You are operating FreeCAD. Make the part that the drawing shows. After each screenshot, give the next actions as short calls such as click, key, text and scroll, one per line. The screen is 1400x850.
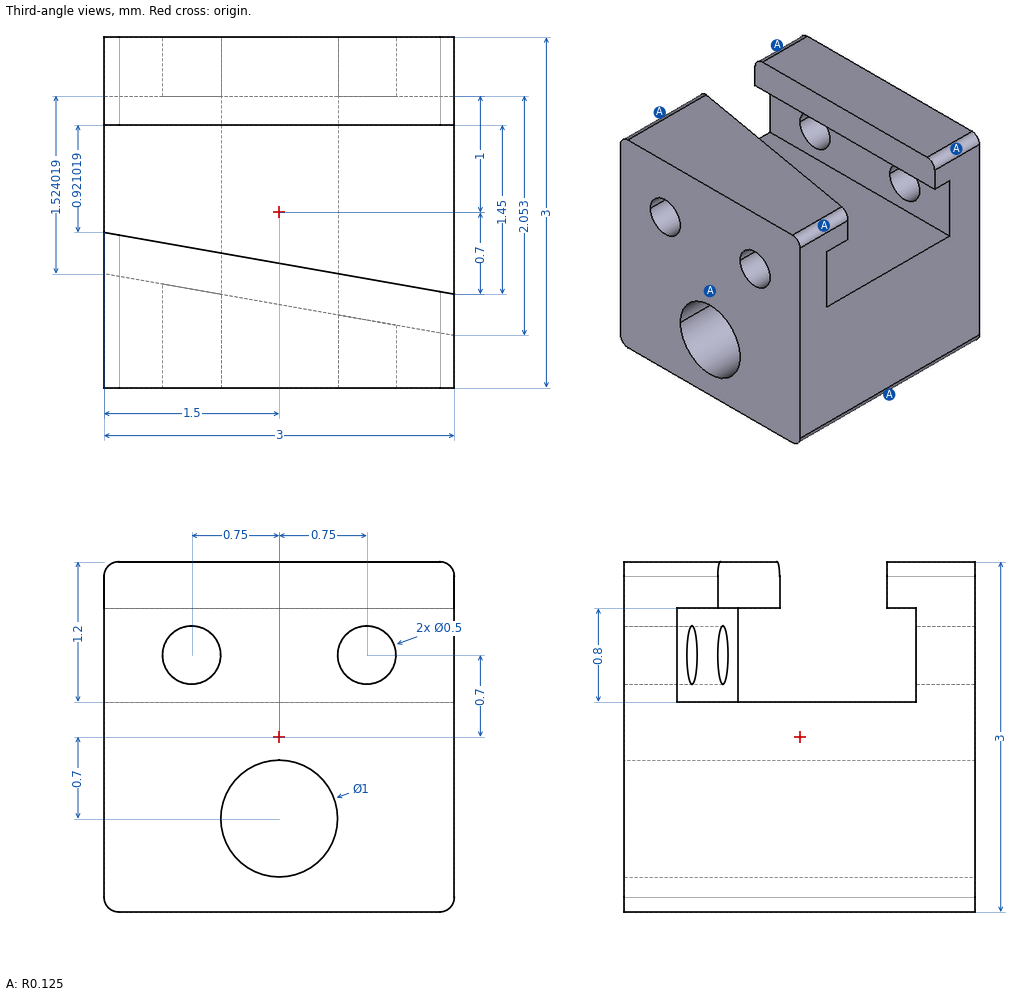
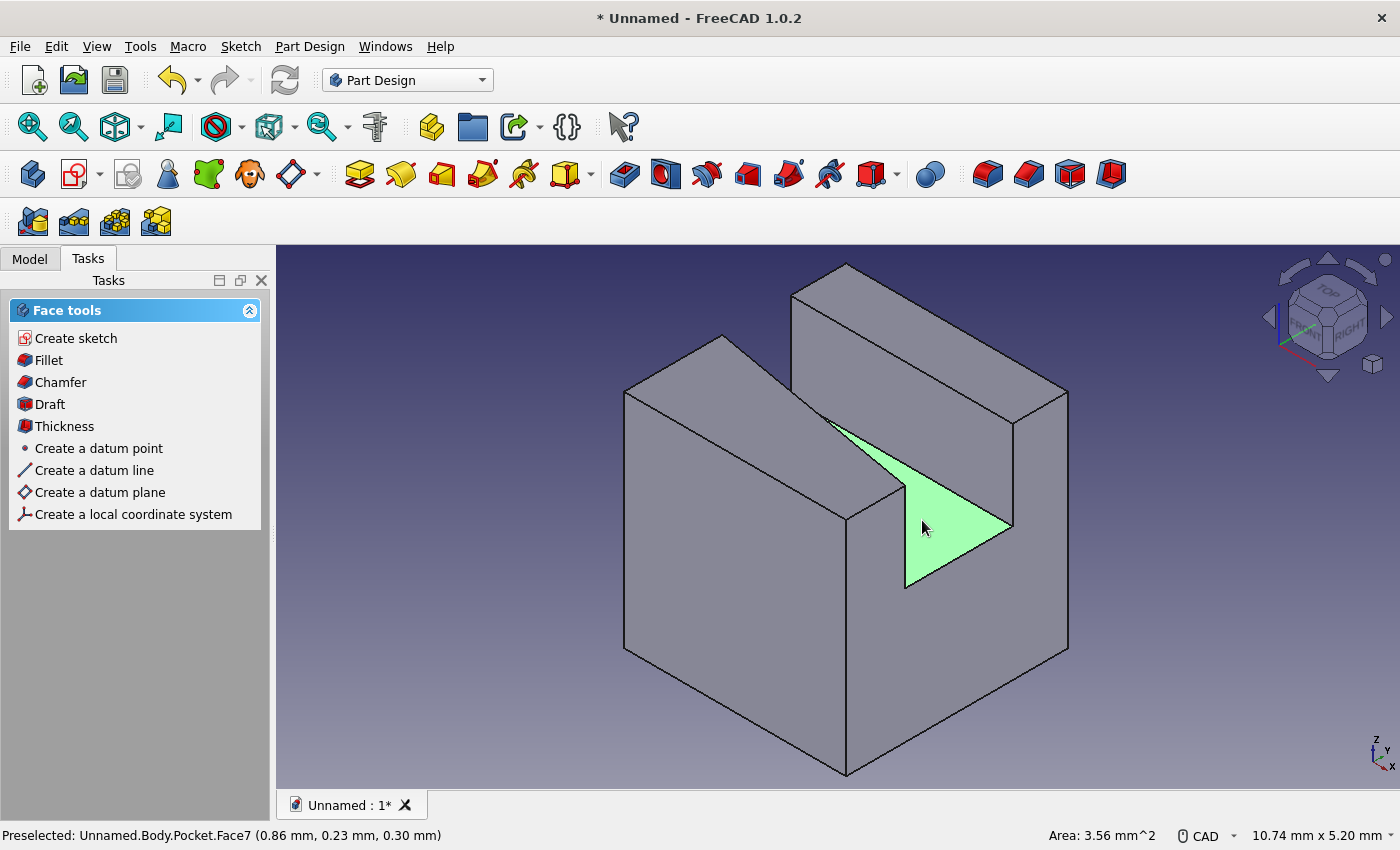
click(74, 174)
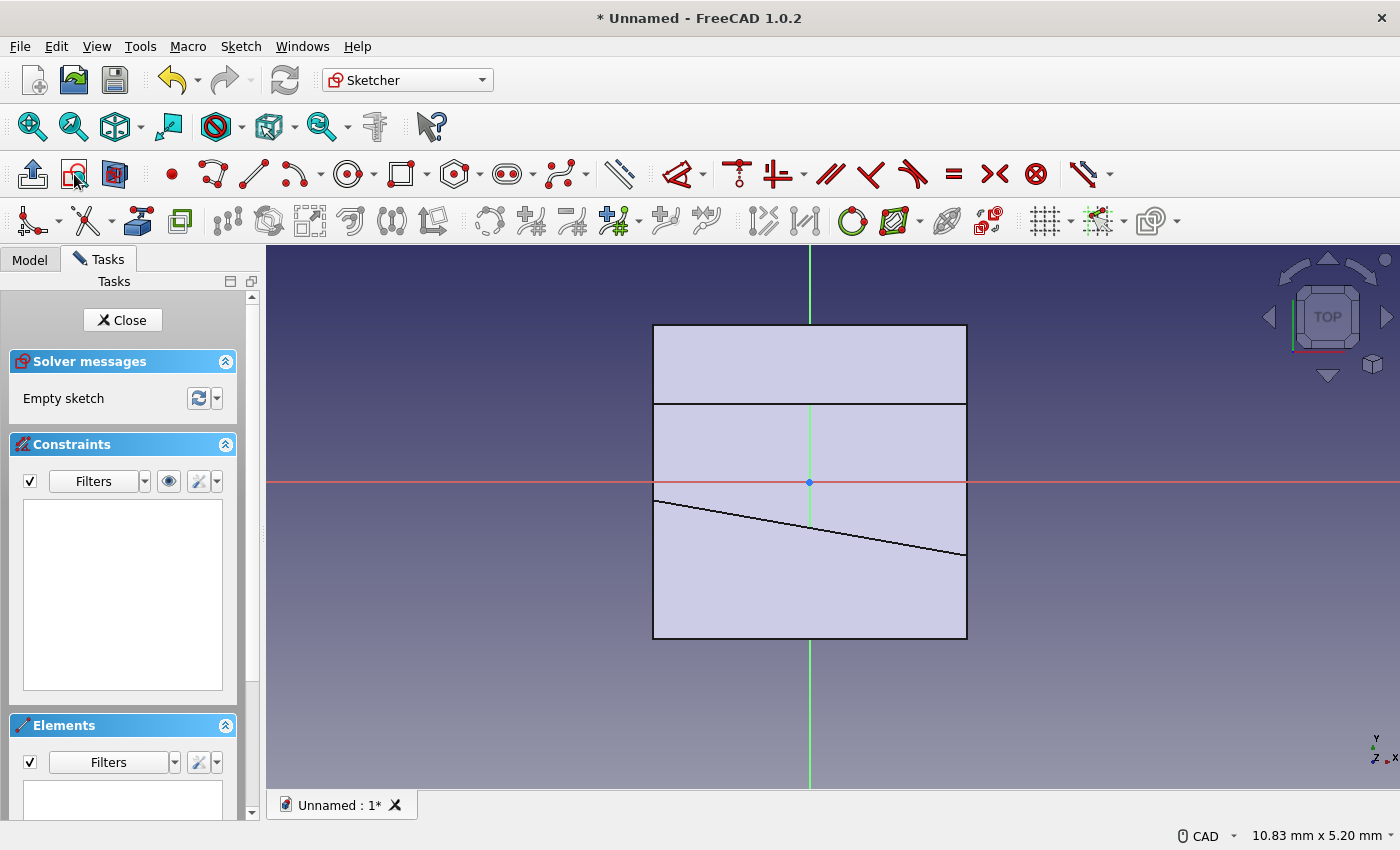
key(q)
key(s)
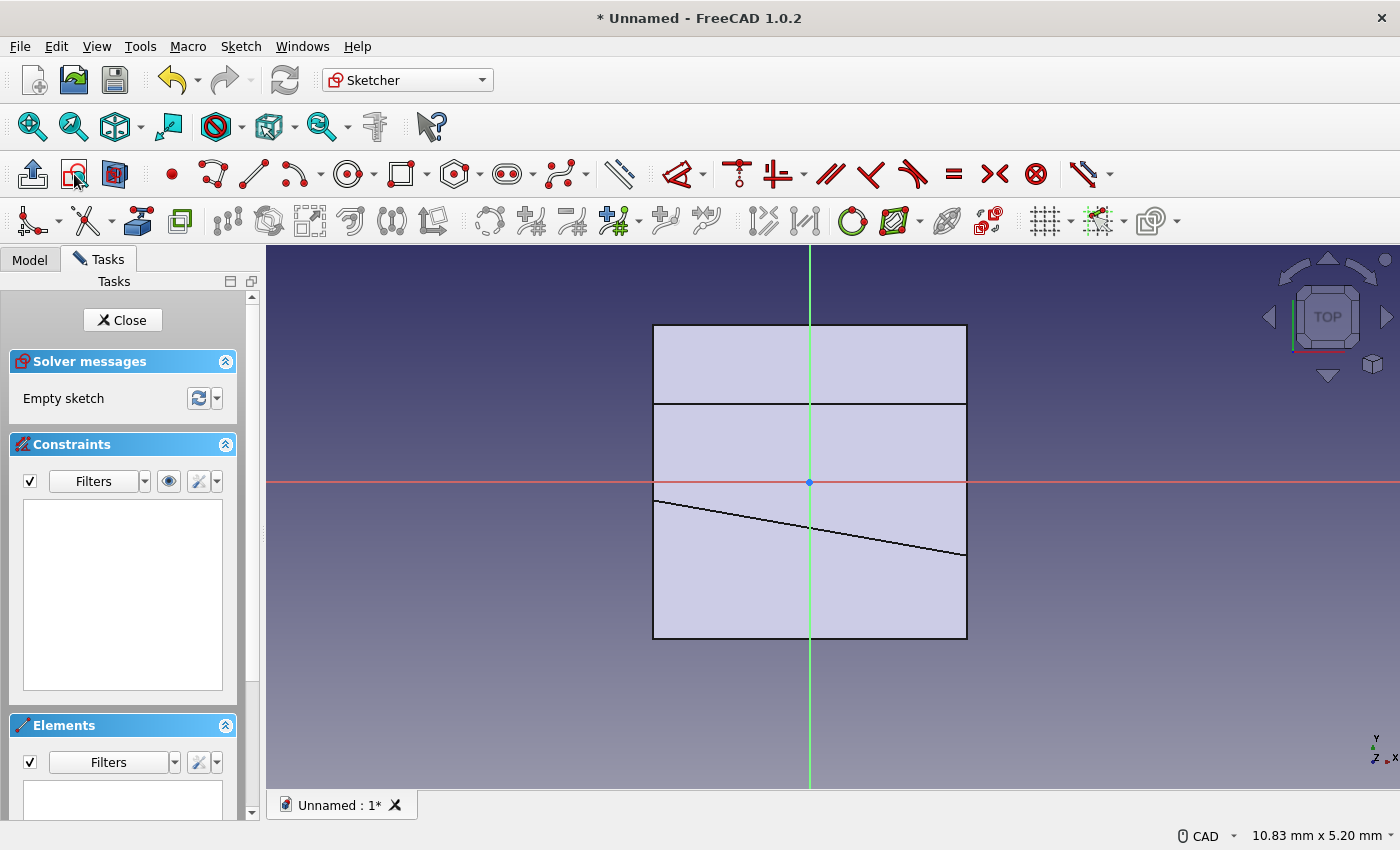
scroll(902, 421, up, 2)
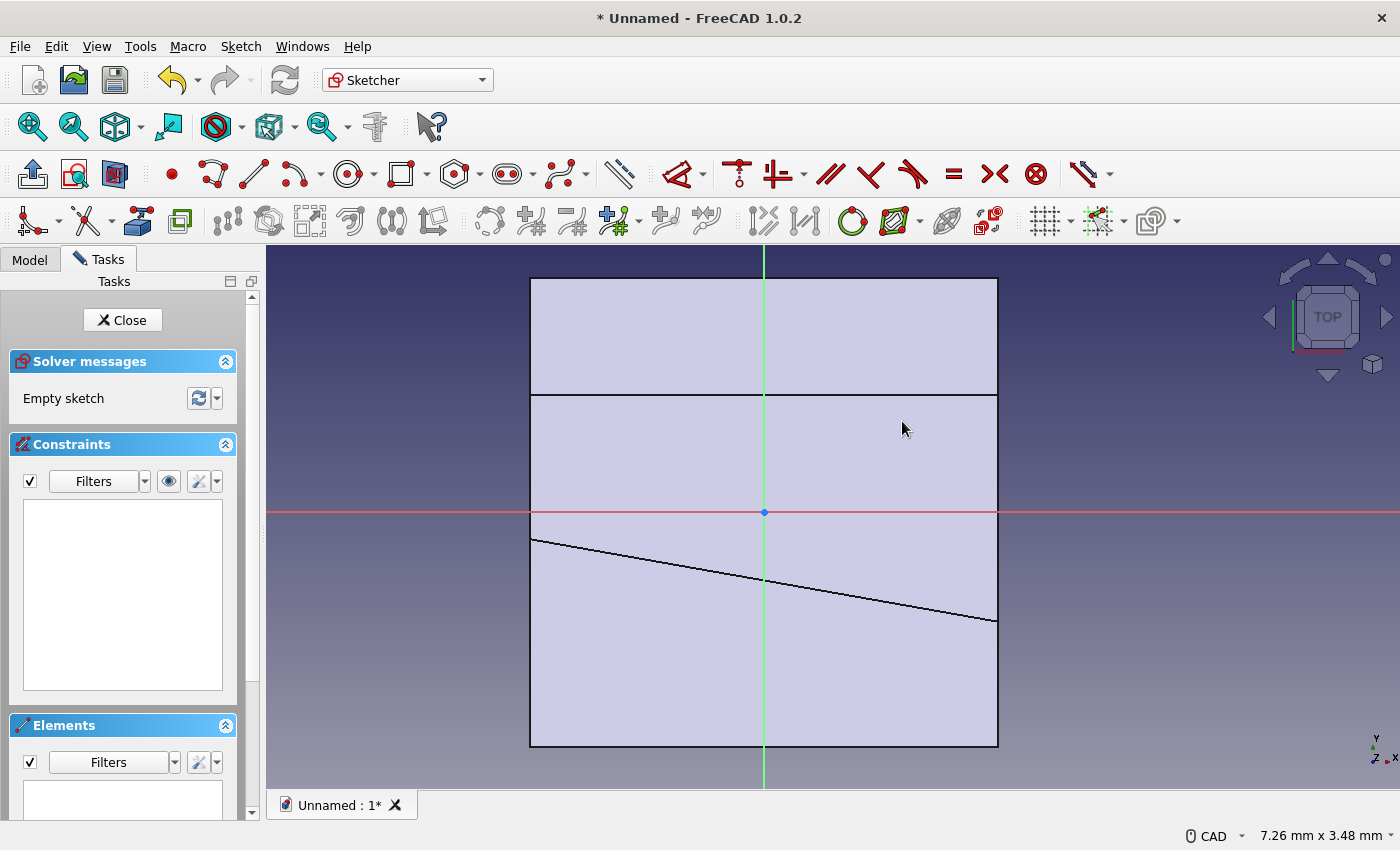
key(g)
key(m)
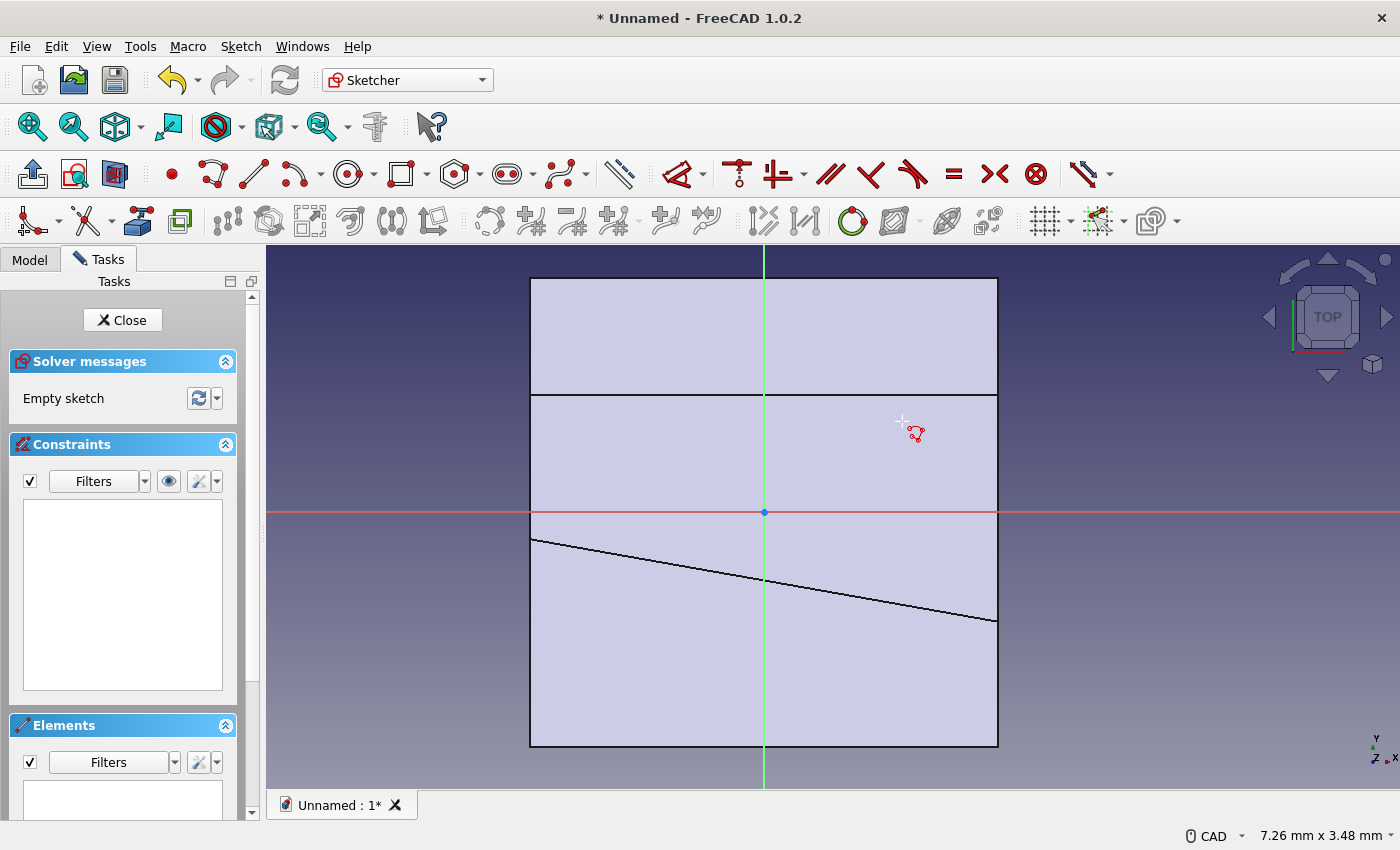
click(530, 594)
click(998, 677)
click(998, 356)
click(530, 356)
click(530, 595)
key(Escape)
key(Escape)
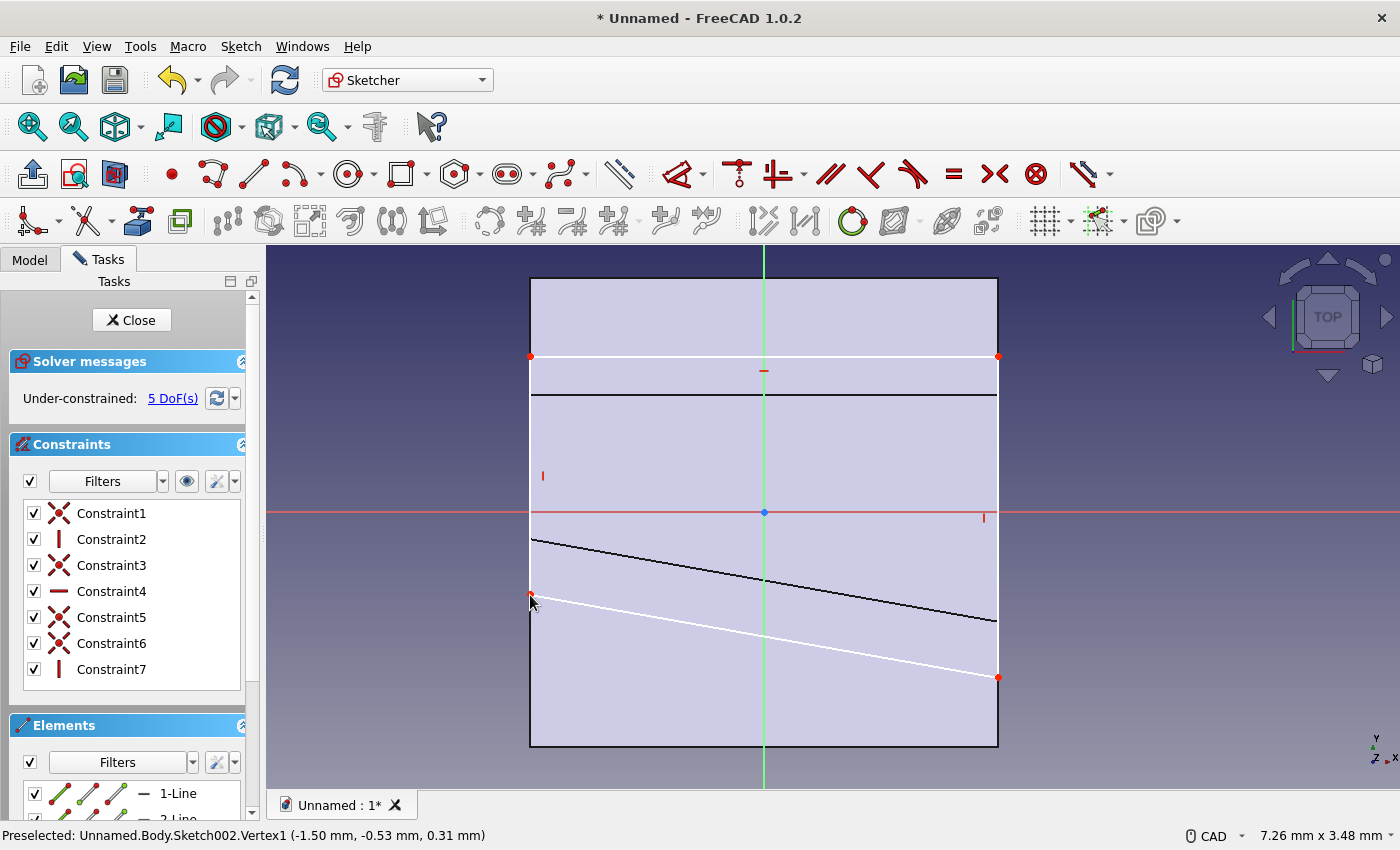
key(d)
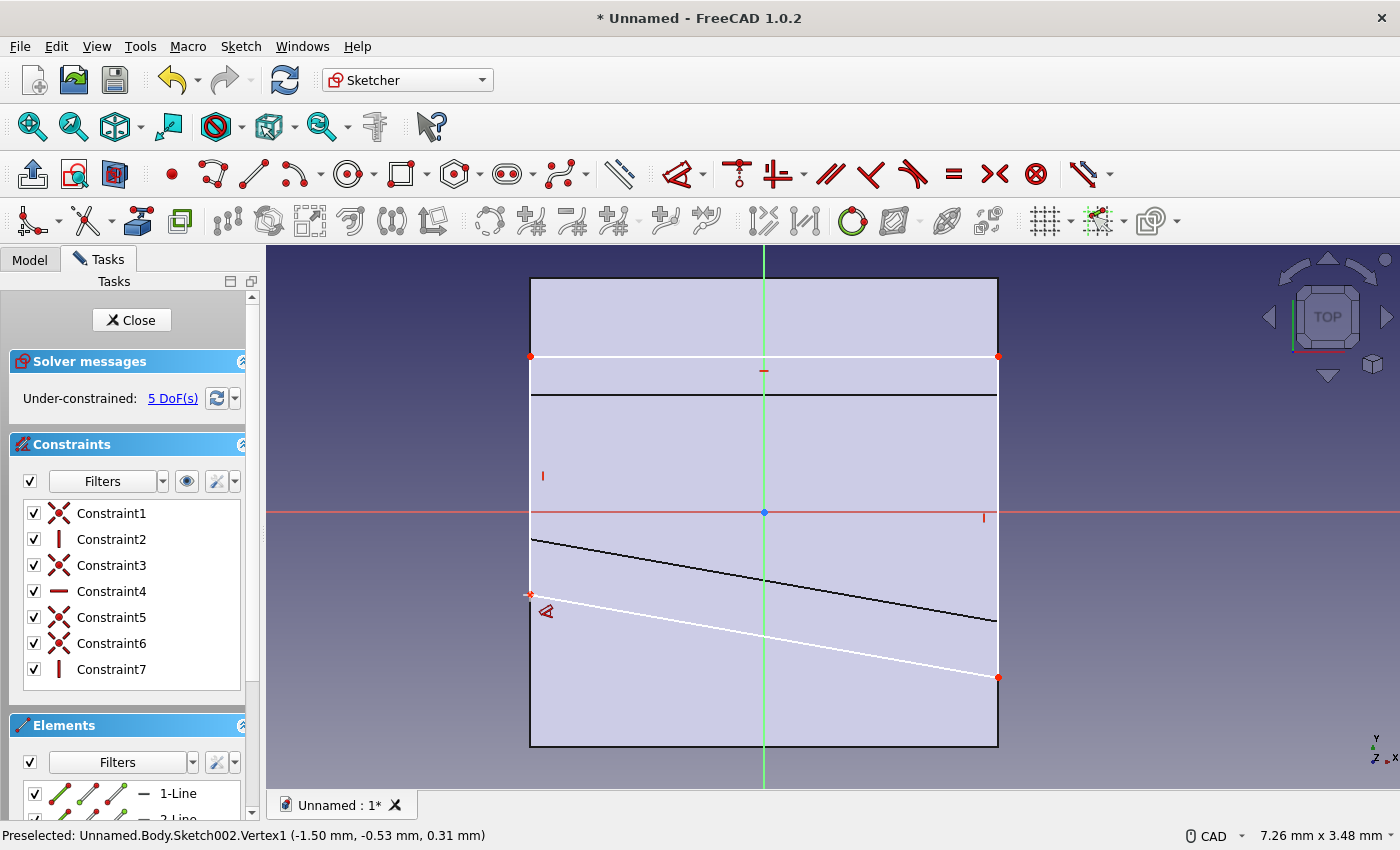
click(858, 357)
click(656, 323)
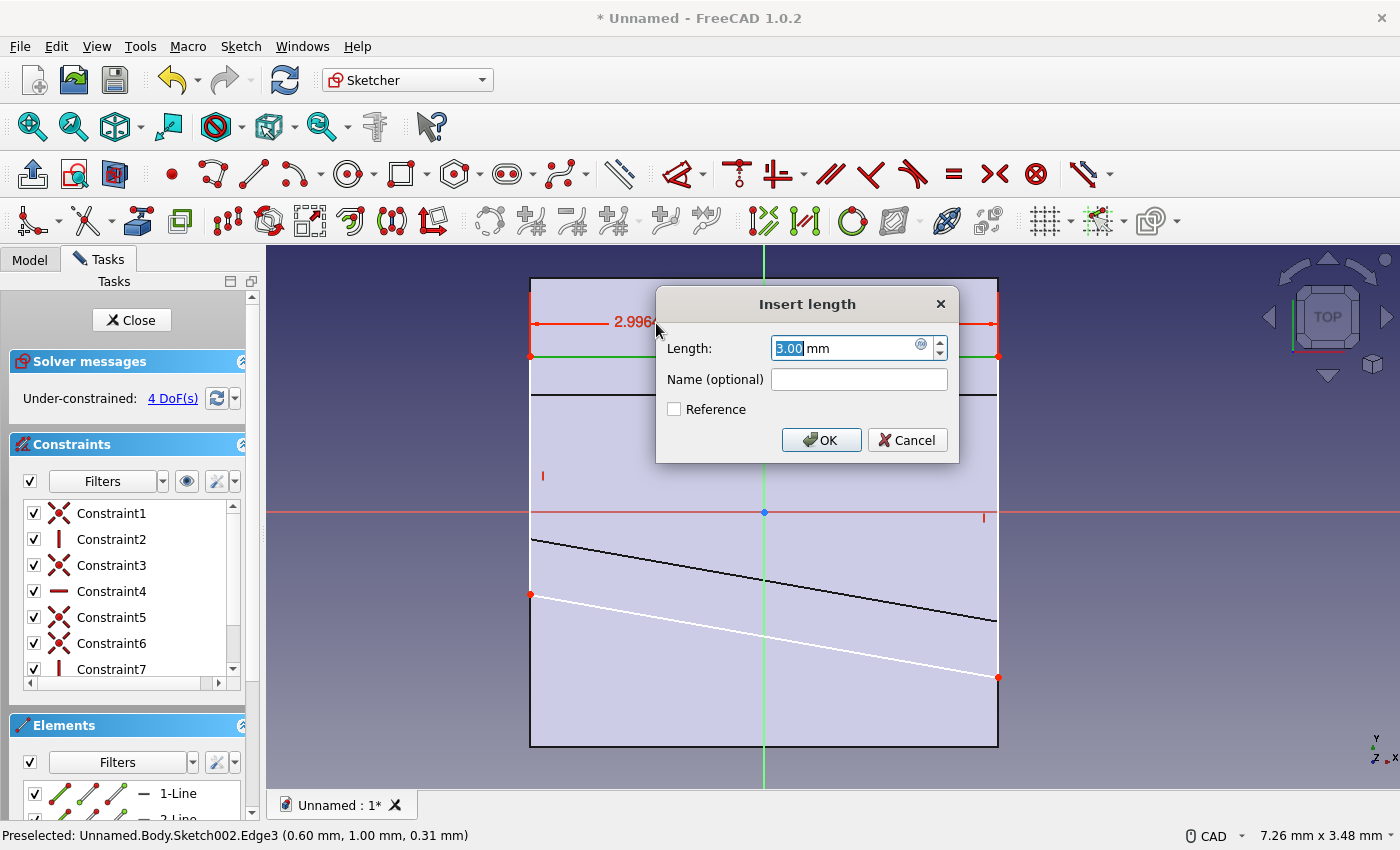
text(3)
key(Return)